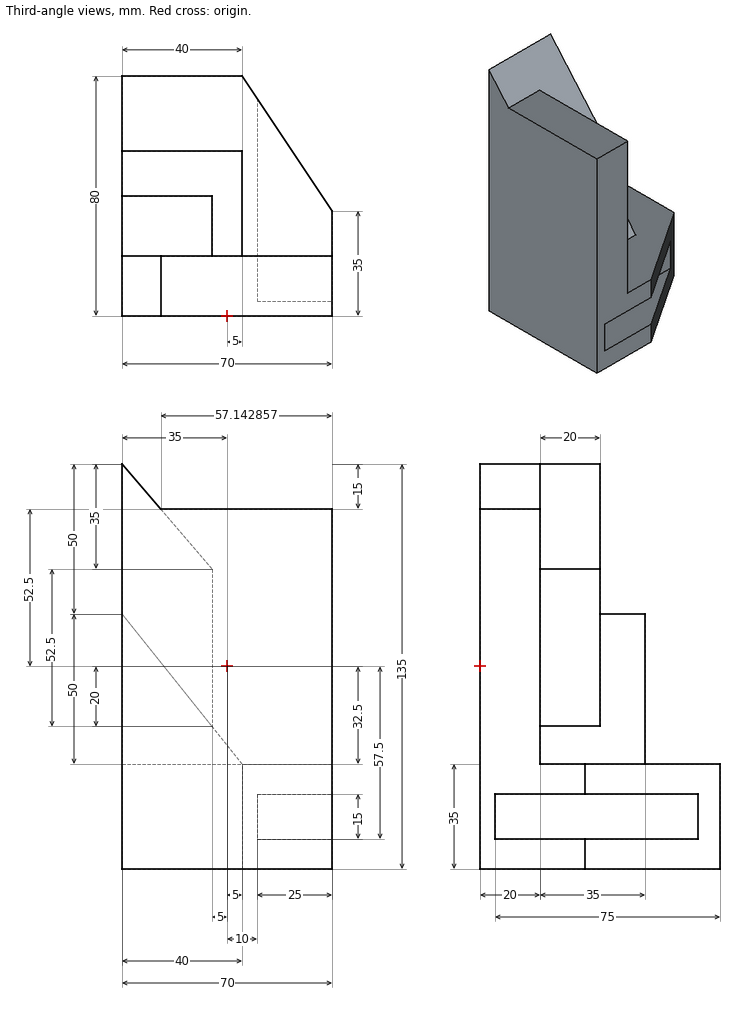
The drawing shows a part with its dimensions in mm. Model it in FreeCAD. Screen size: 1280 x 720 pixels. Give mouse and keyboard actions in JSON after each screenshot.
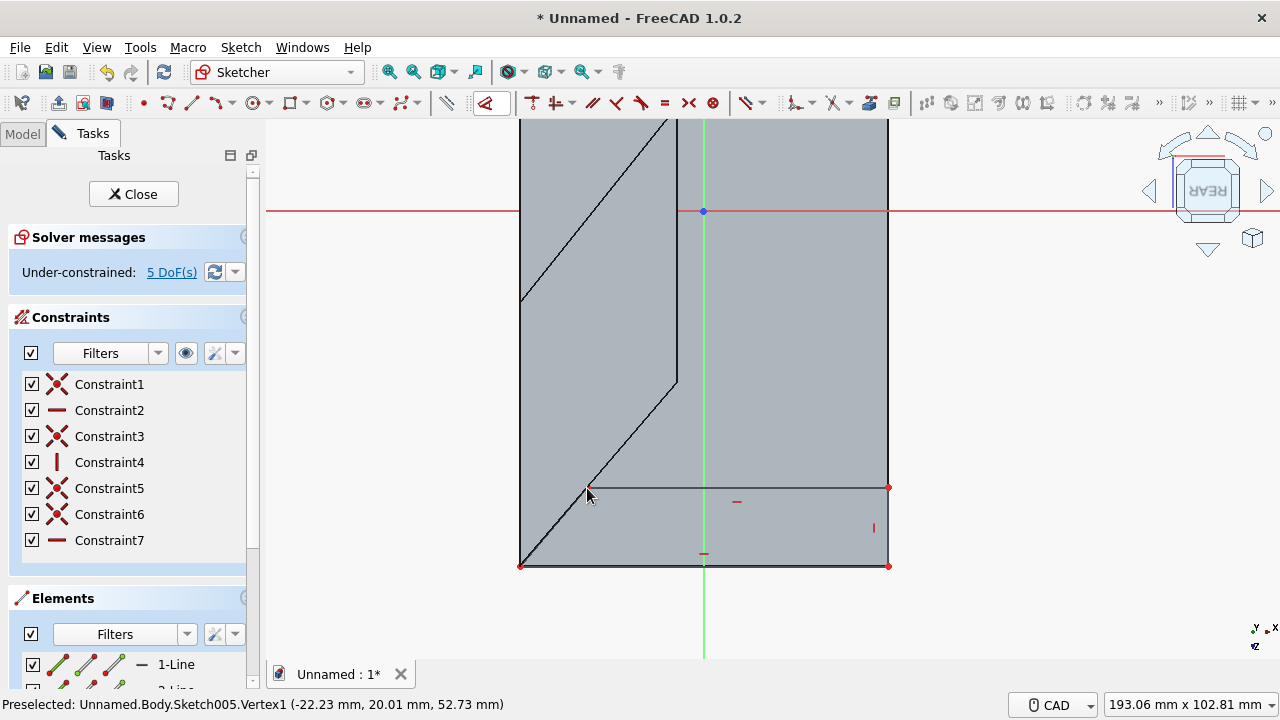
{"action": "left_click", "coordinate": [630, 567]}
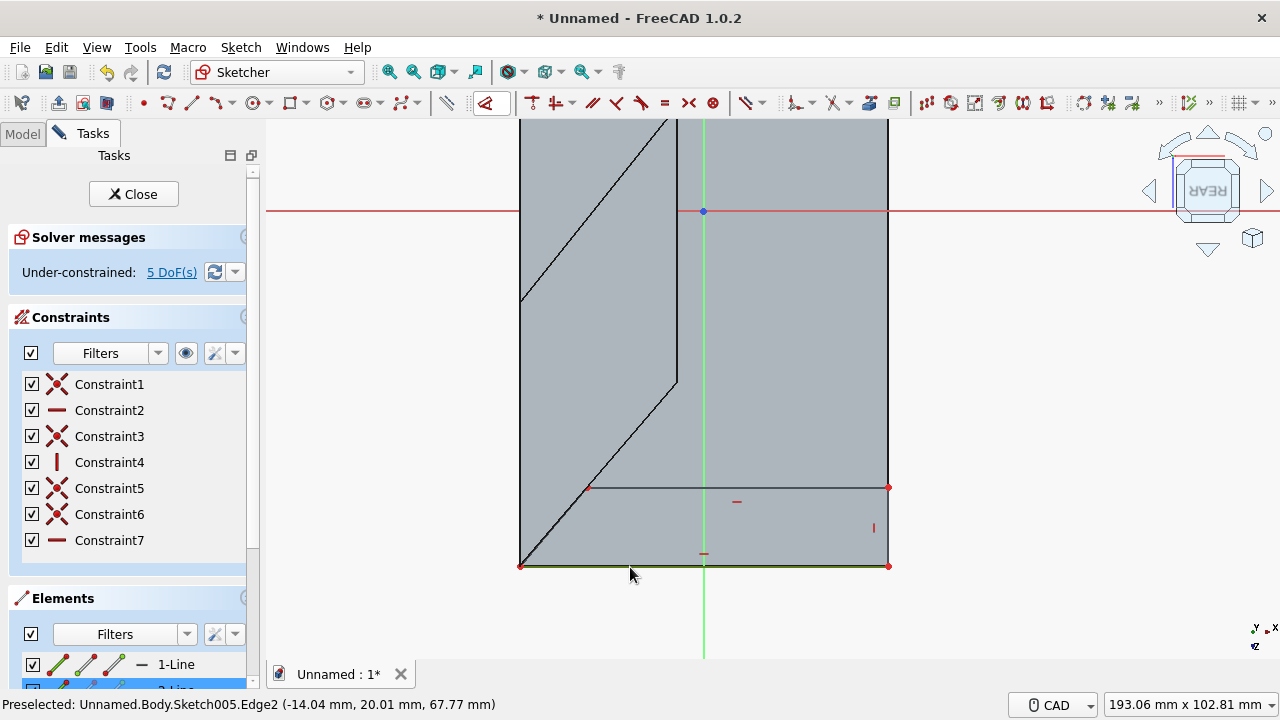
{"action": "key", "text": "l"}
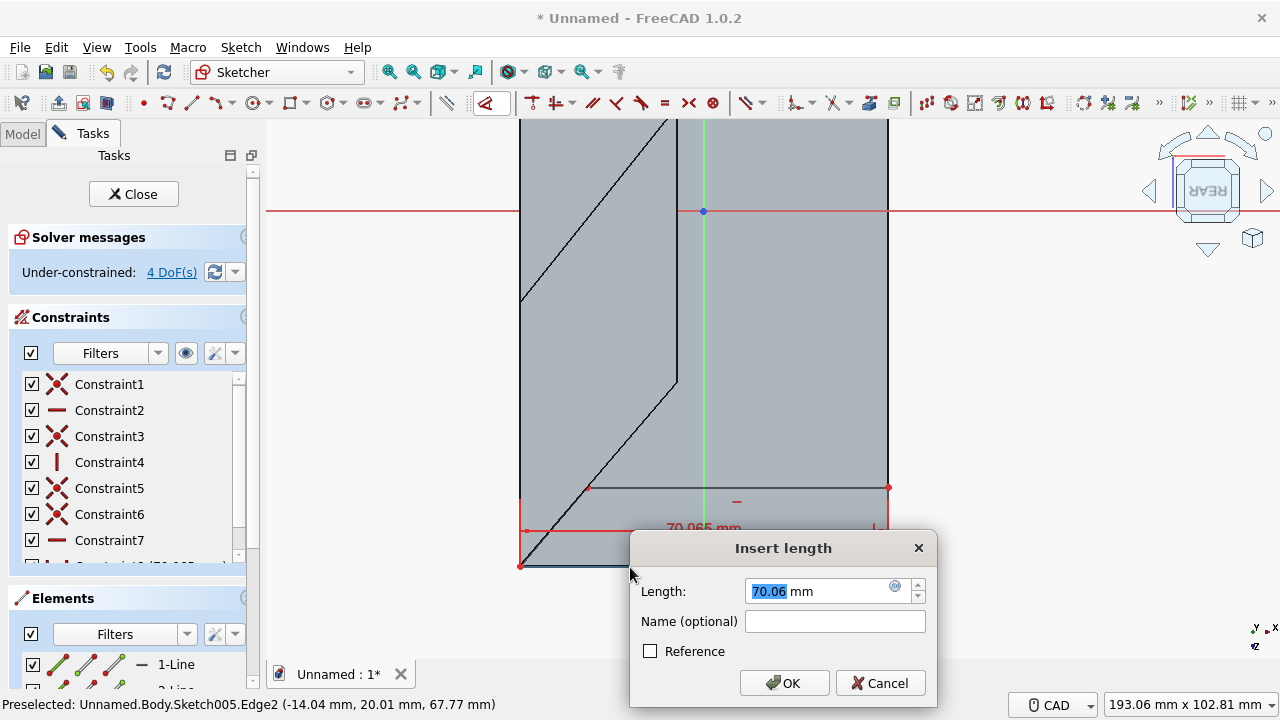
{"action": "type", "text": "70"}
{"action": "key", "text": "Return"}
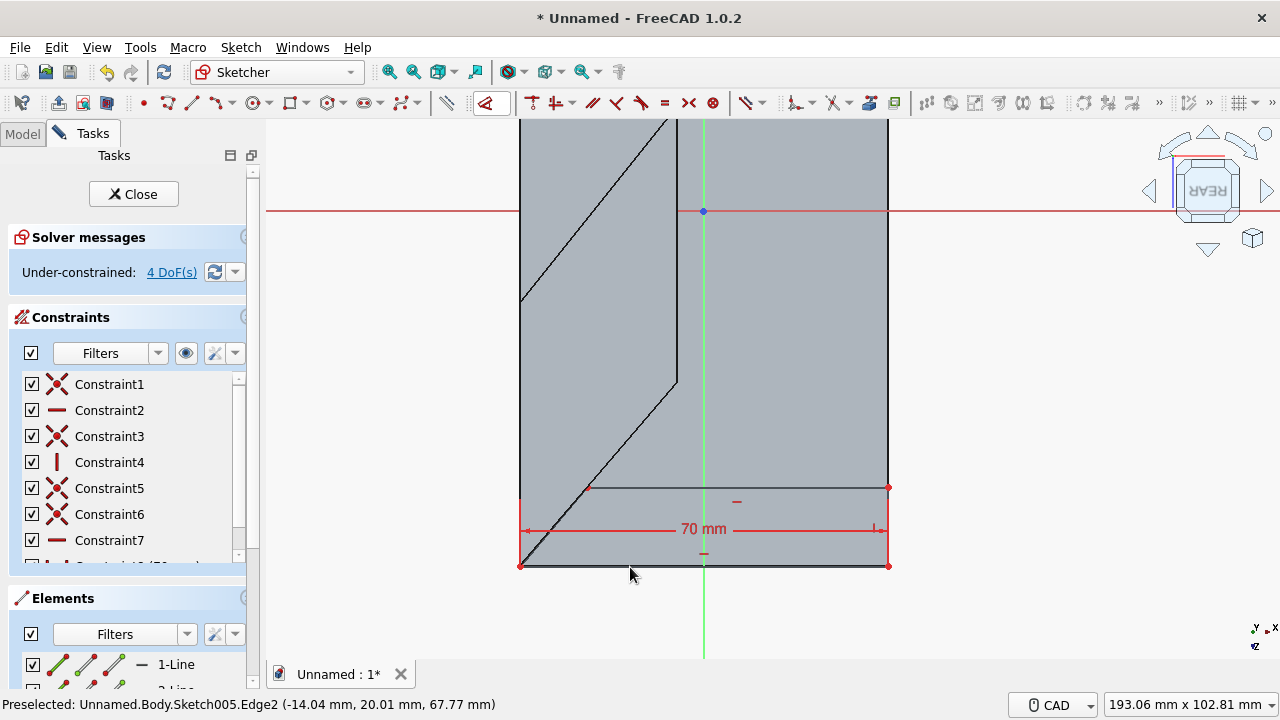
{"action": "left_click", "coordinate": [888, 543]}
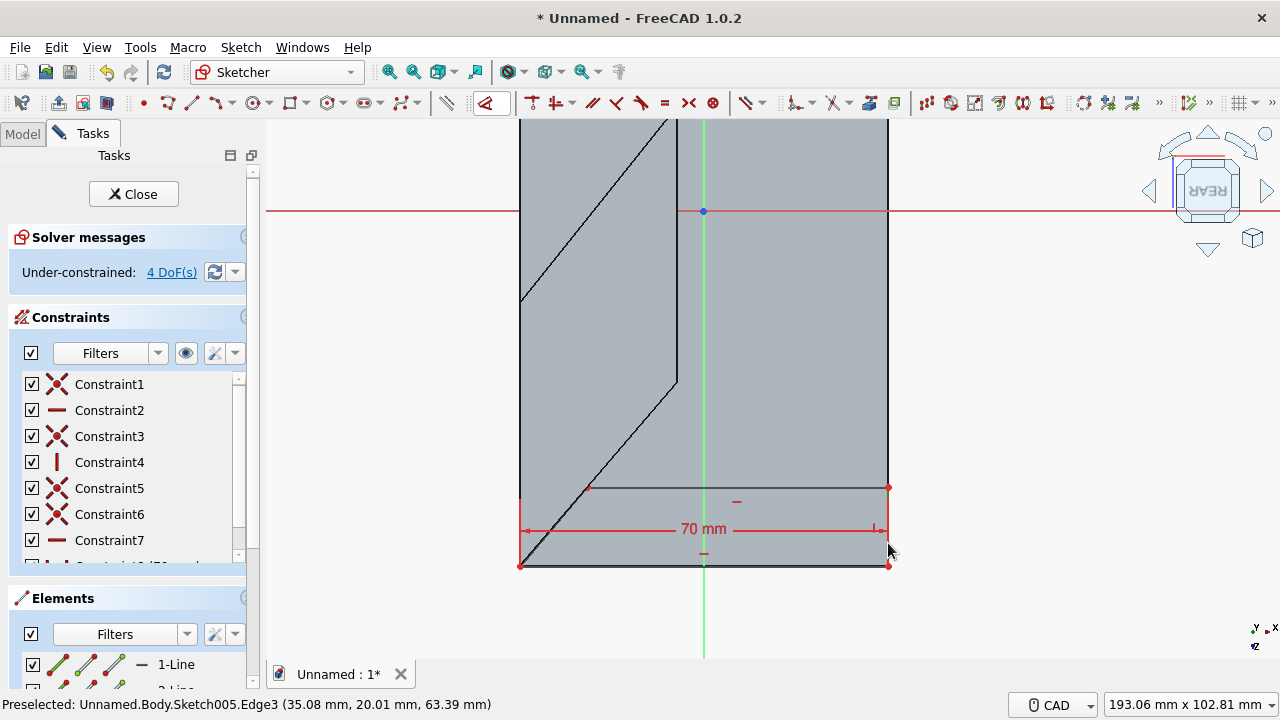
{"action": "left_click", "coordinate": [504, 104]}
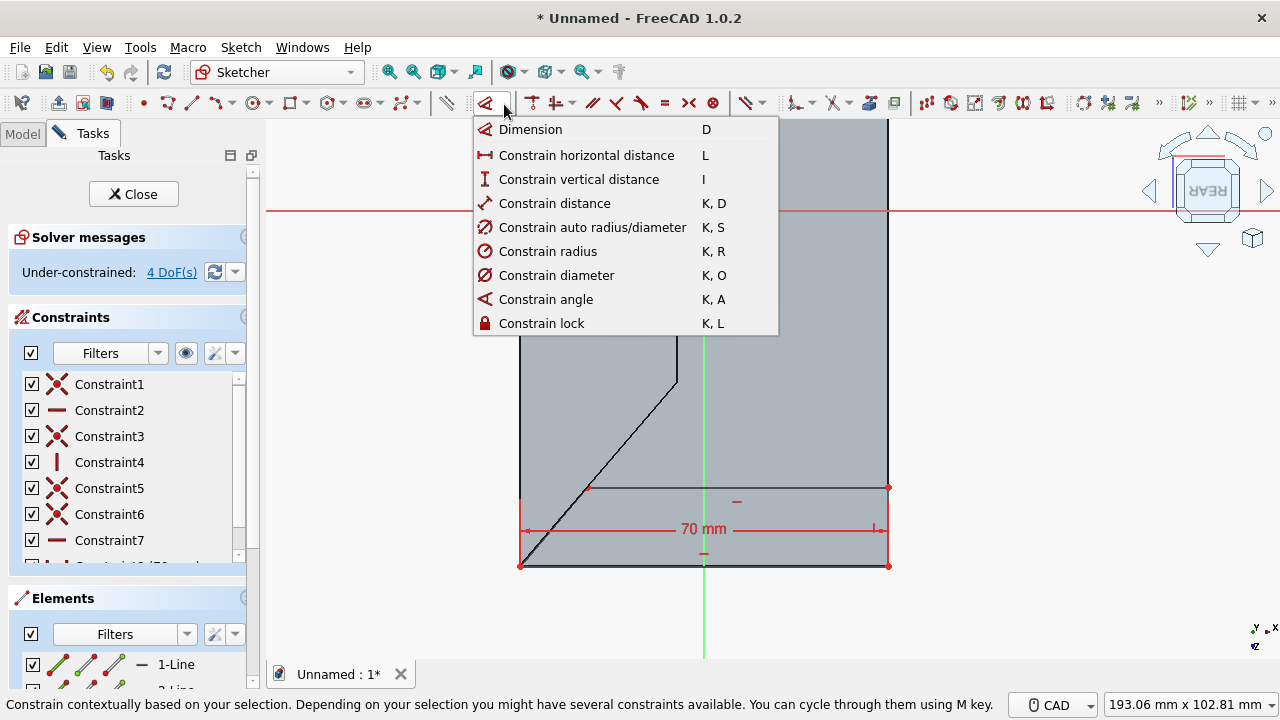
{"action": "left_click", "coordinate": [626, 179]}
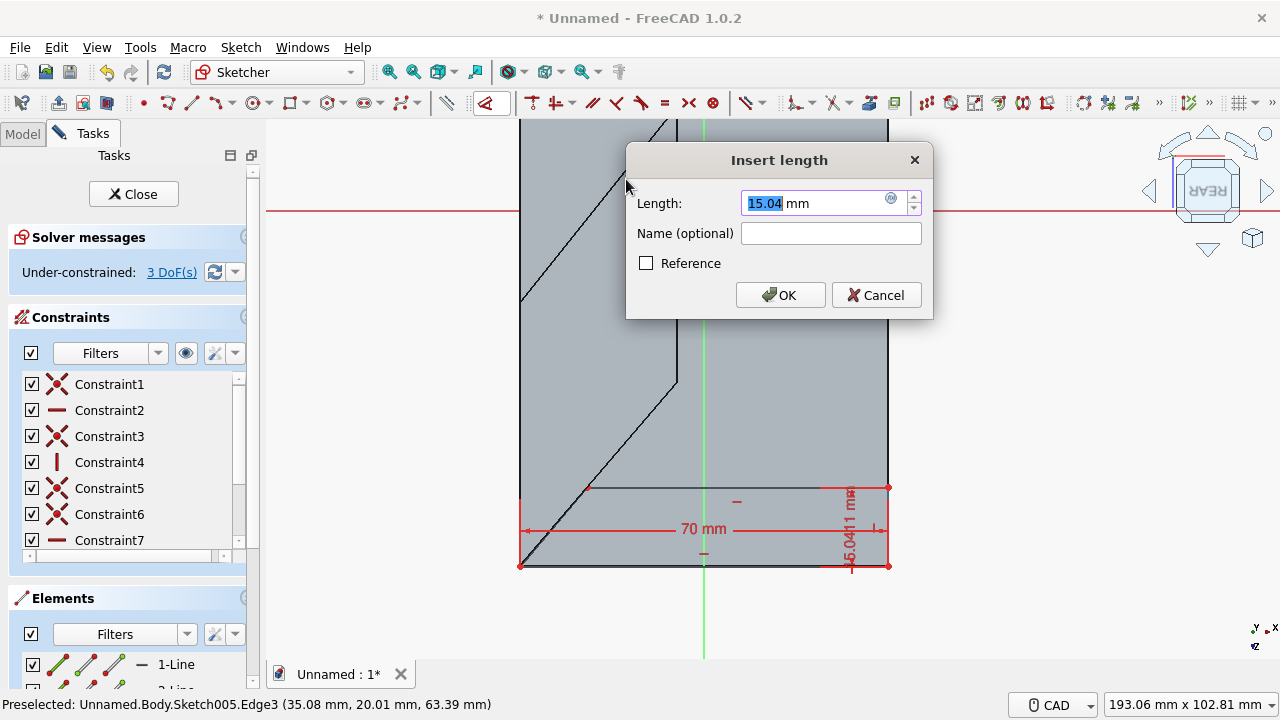
{"action": "type", "text": "15"}
{"action": "key", "text": "Return"}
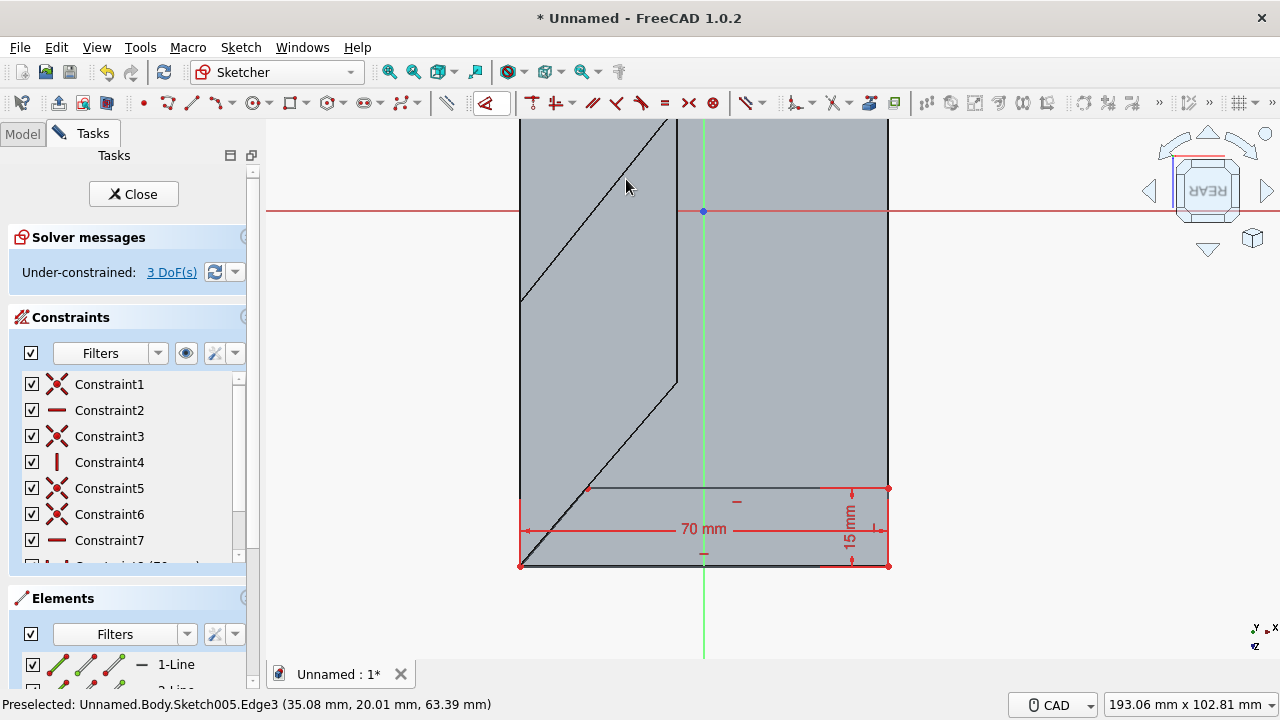
{"action": "left_click", "coordinate": [520, 567]}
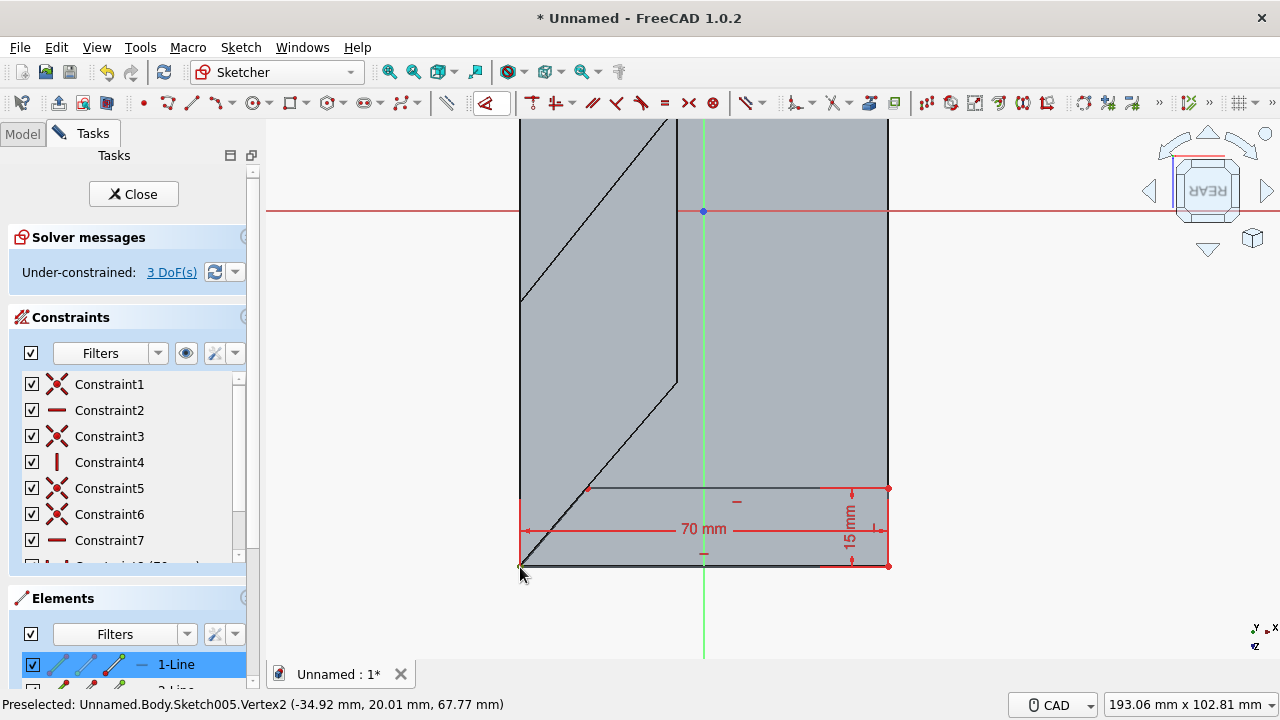
{"action": "left_click", "coordinate": [504, 104]}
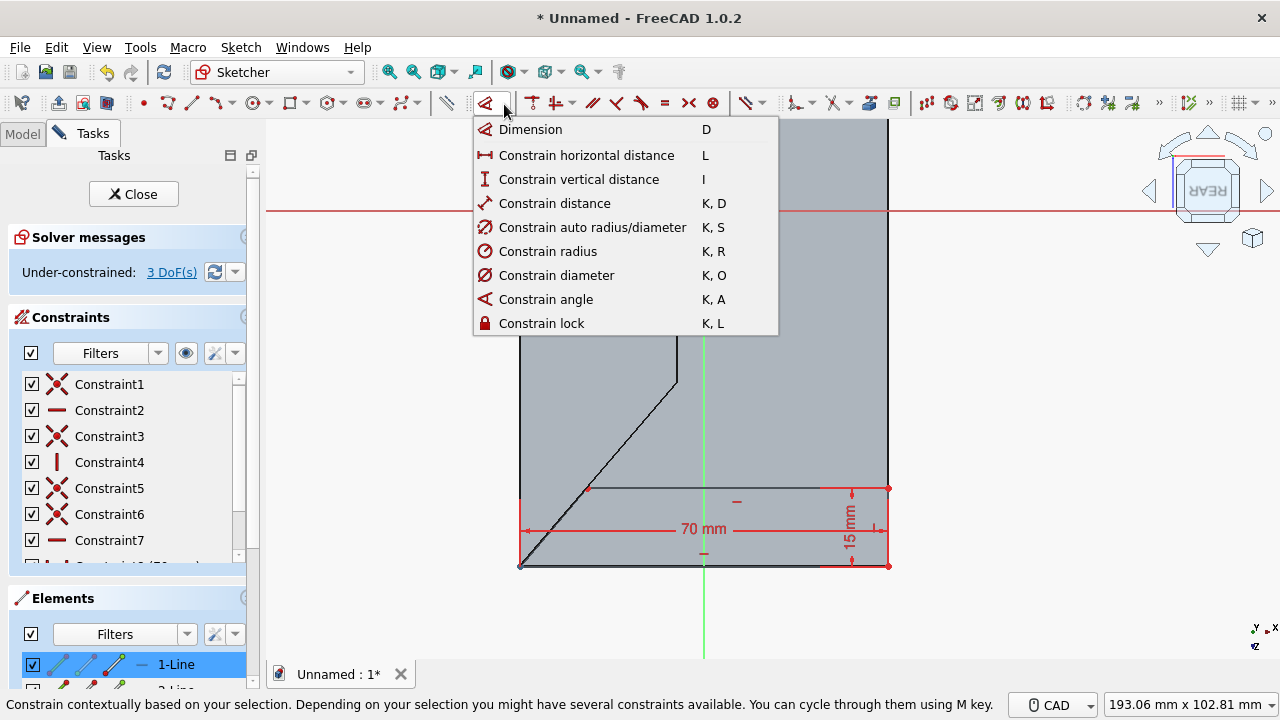
{"action": "left_click", "coordinate": [626, 155]}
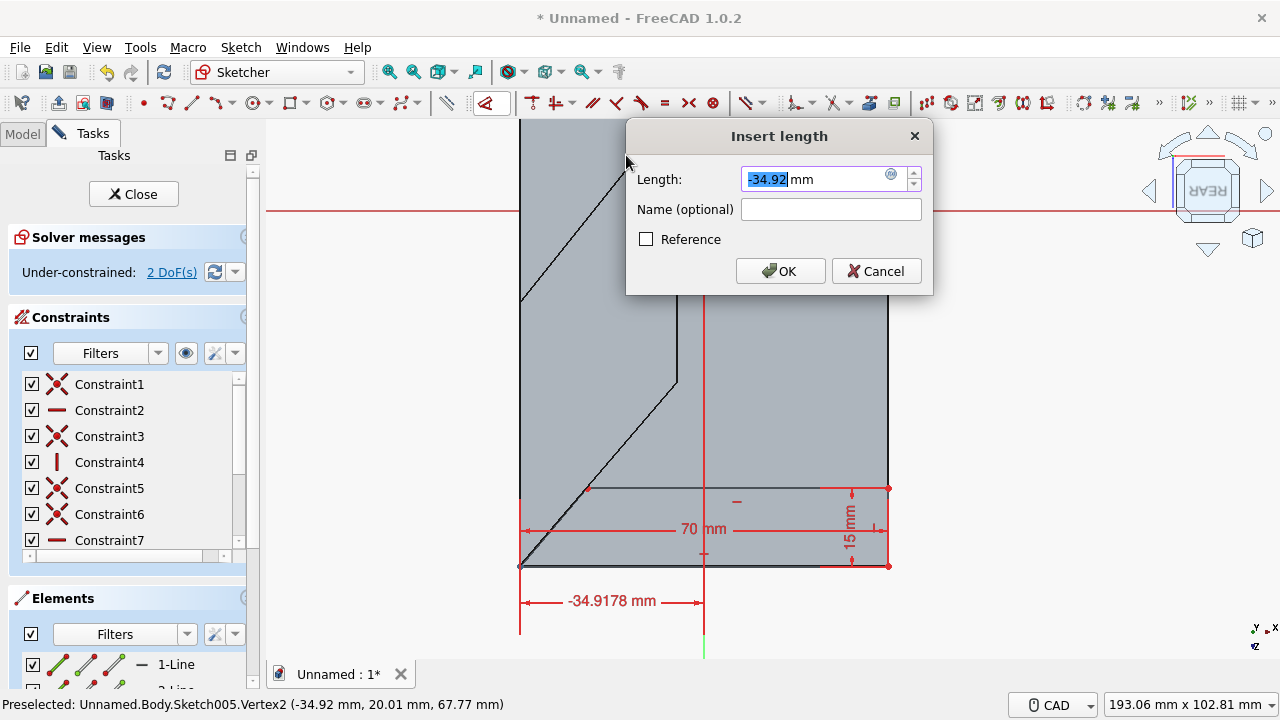
{"action": "type", "text": "-35"}
{"action": "key", "text": "Return"}